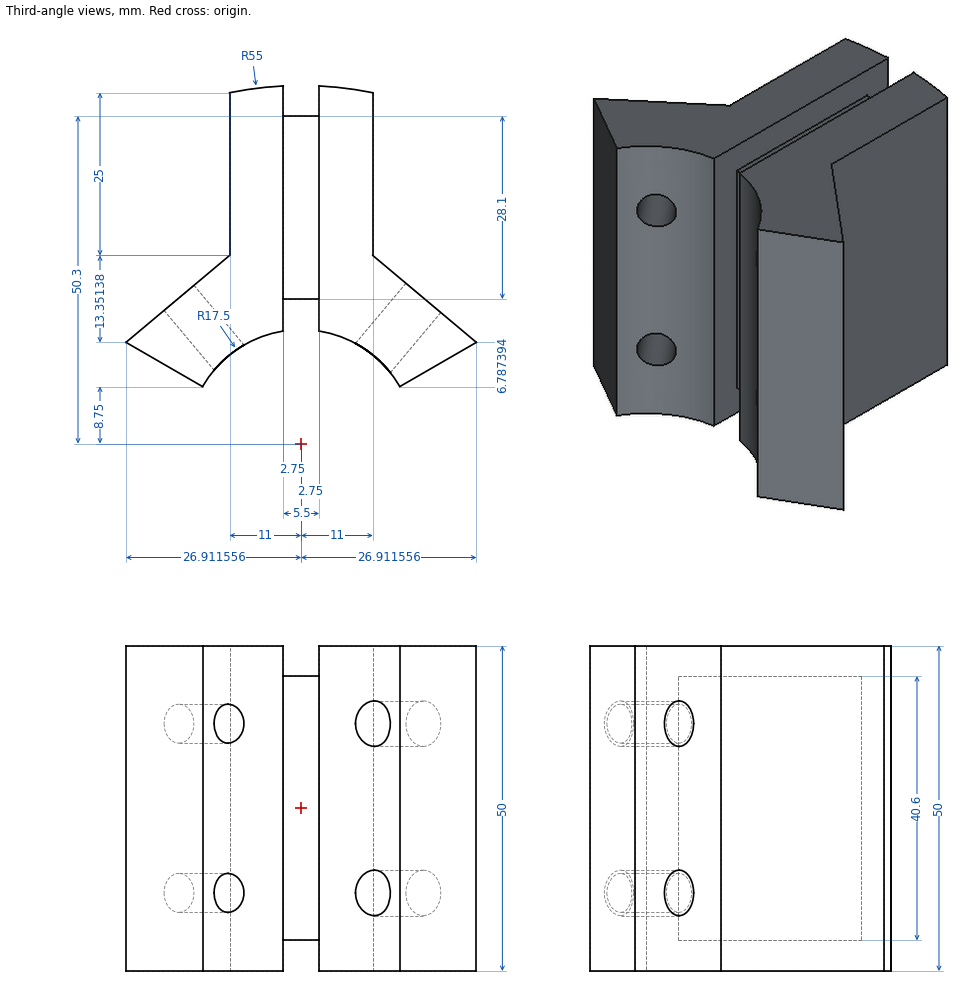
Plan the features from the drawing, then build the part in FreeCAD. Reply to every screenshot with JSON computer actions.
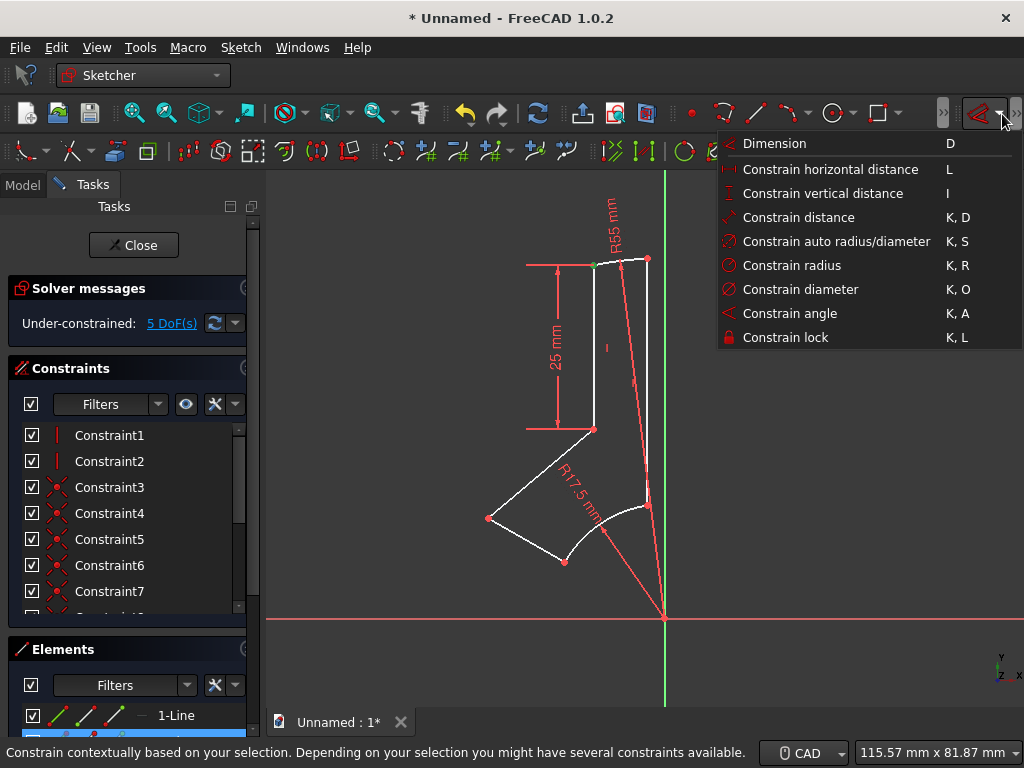
{"action": "left_click", "coordinate": [870, 169]}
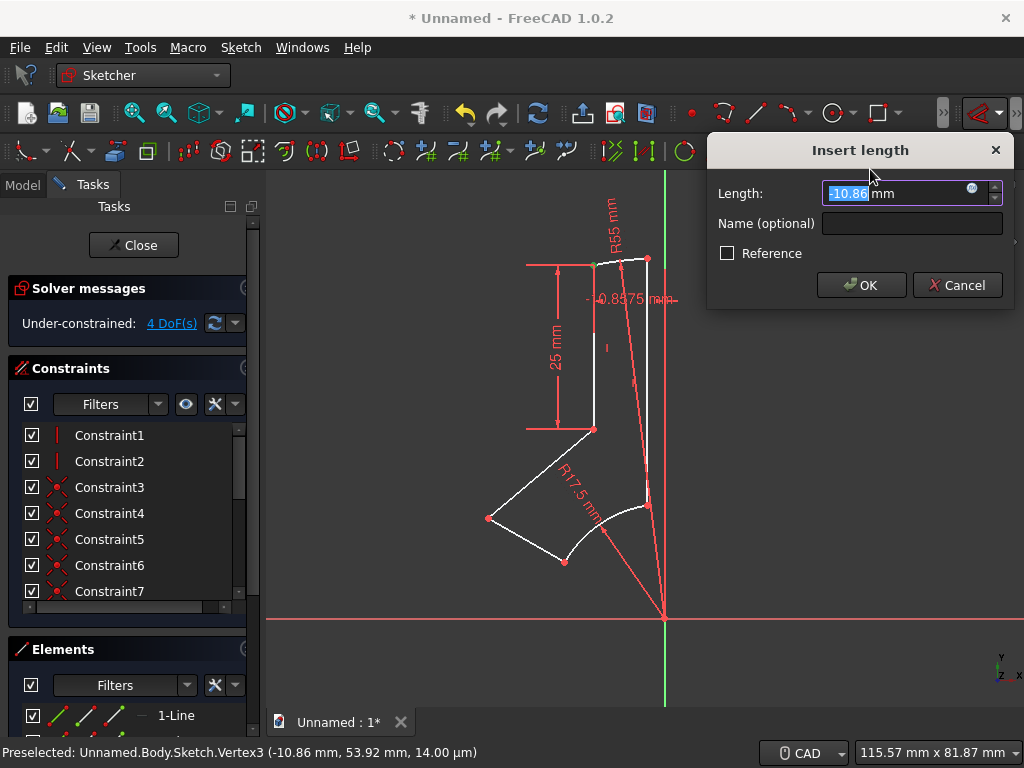
{"action": "type", "text": "-11"}
{"action": "key", "text": "Return"}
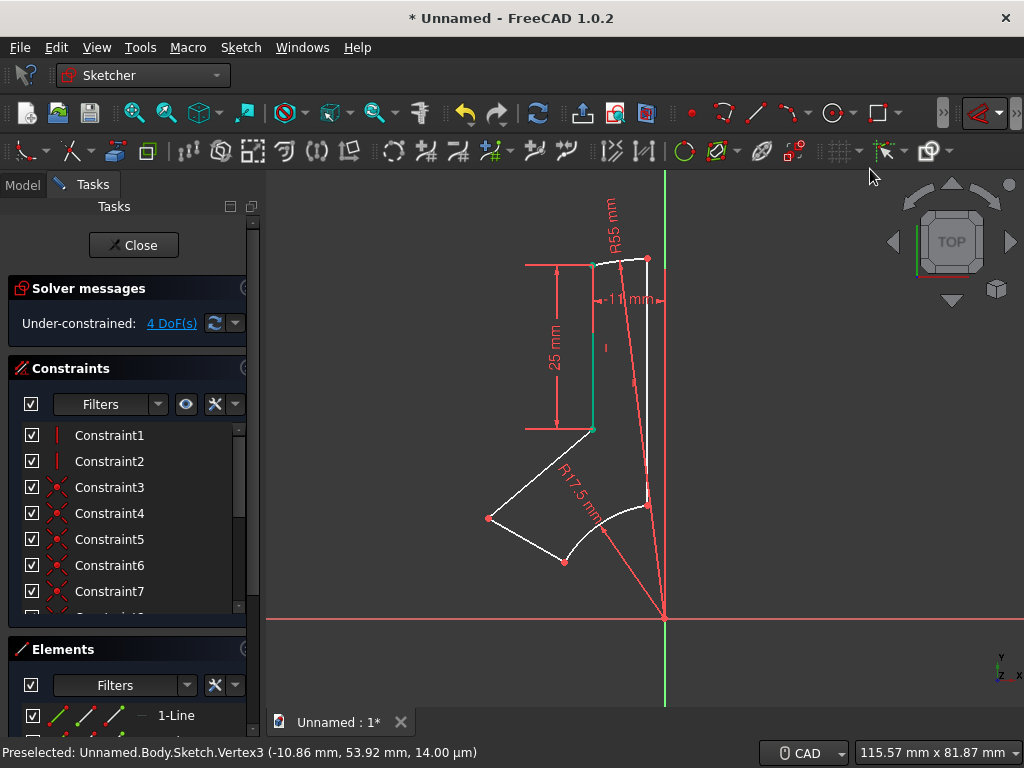
{"action": "scroll", "coordinate": [647, 506], "scroll_direction": "up", "scroll_amount": 4}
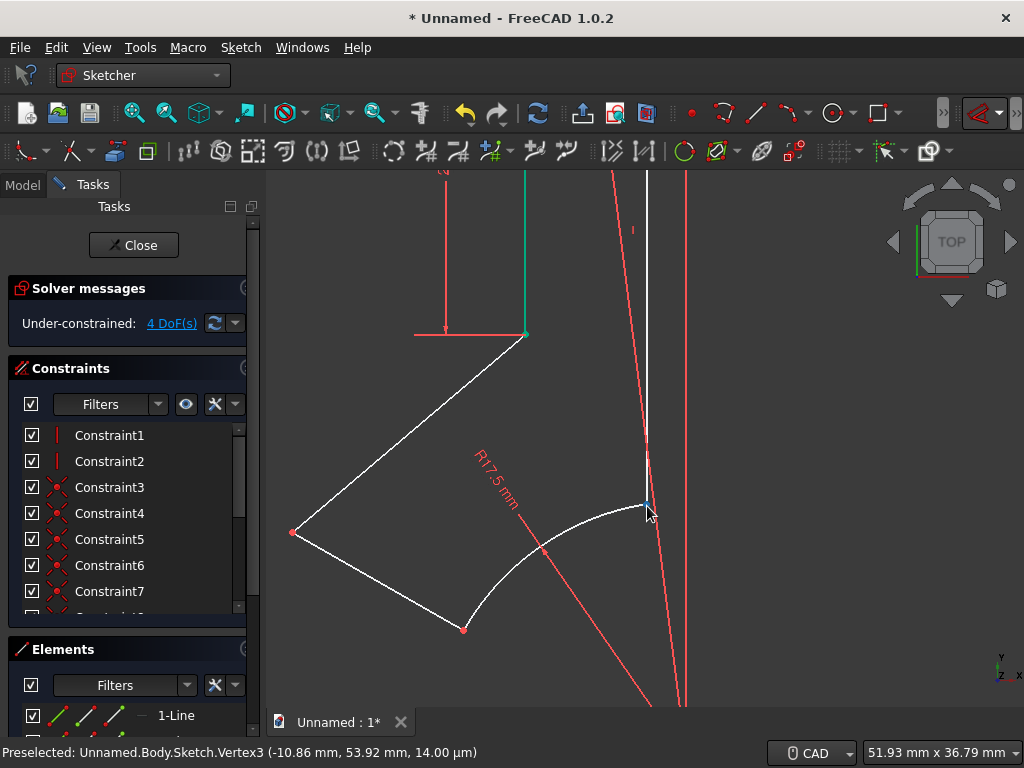
{"action": "left_click", "coordinate": [647, 504]}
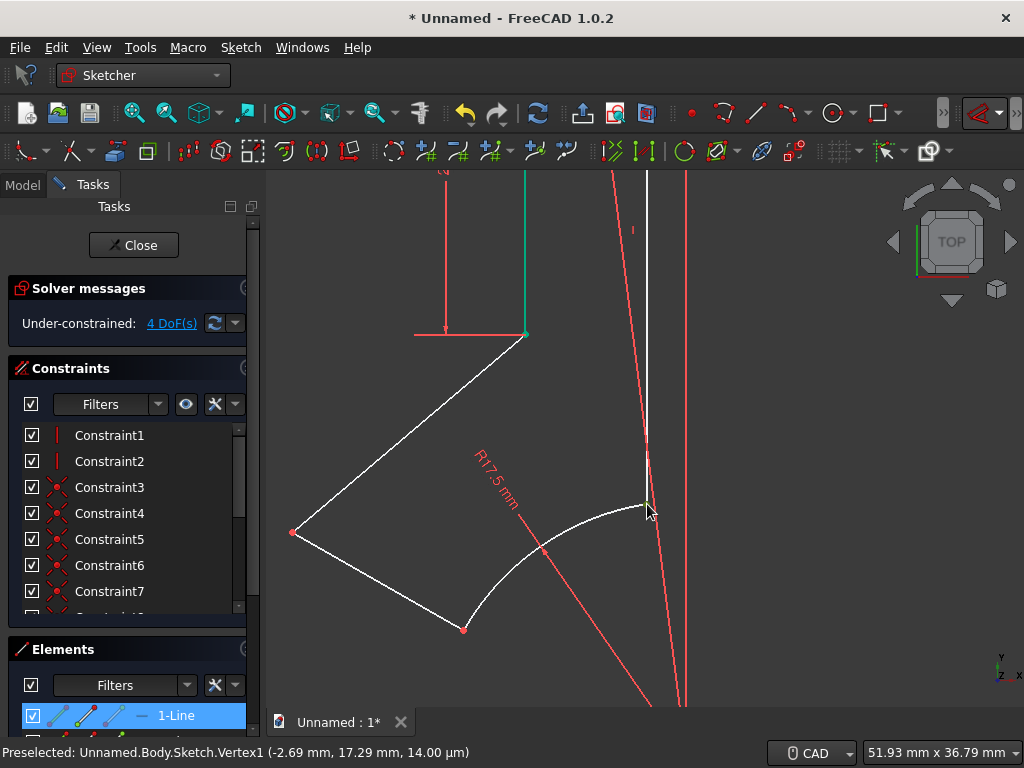
{"action": "key", "text": "l"}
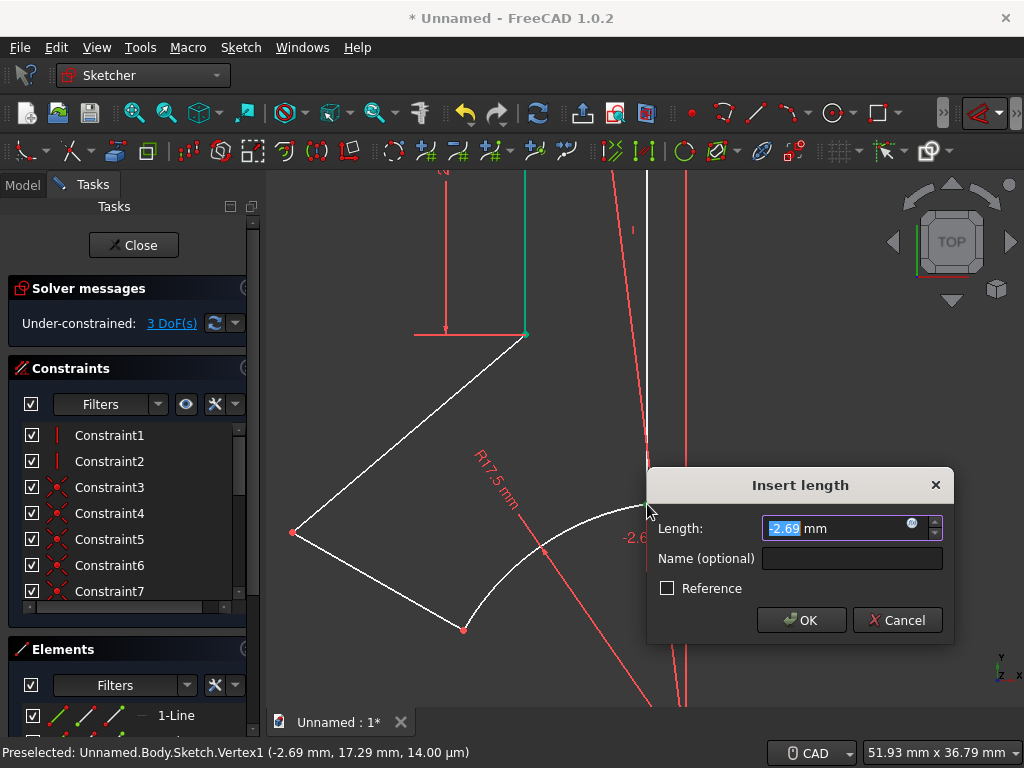
{"action": "type", "text": "-2.75"}
{"action": "key", "text": "Return"}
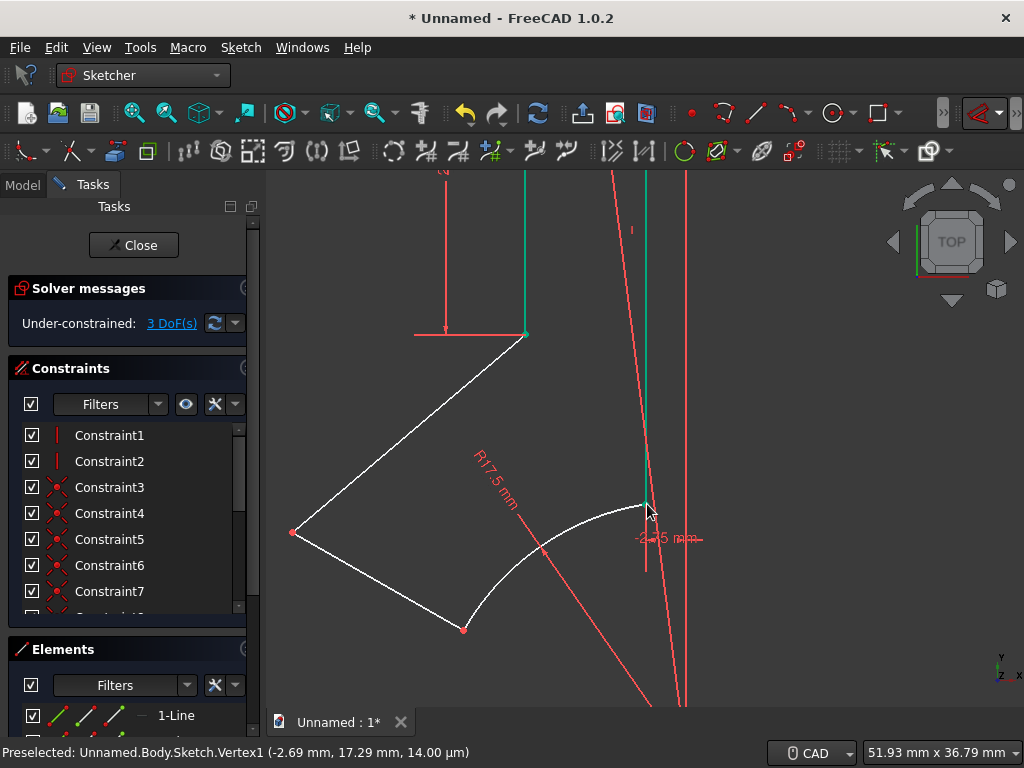
{"action": "left_click", "coordinate": [464, 631]}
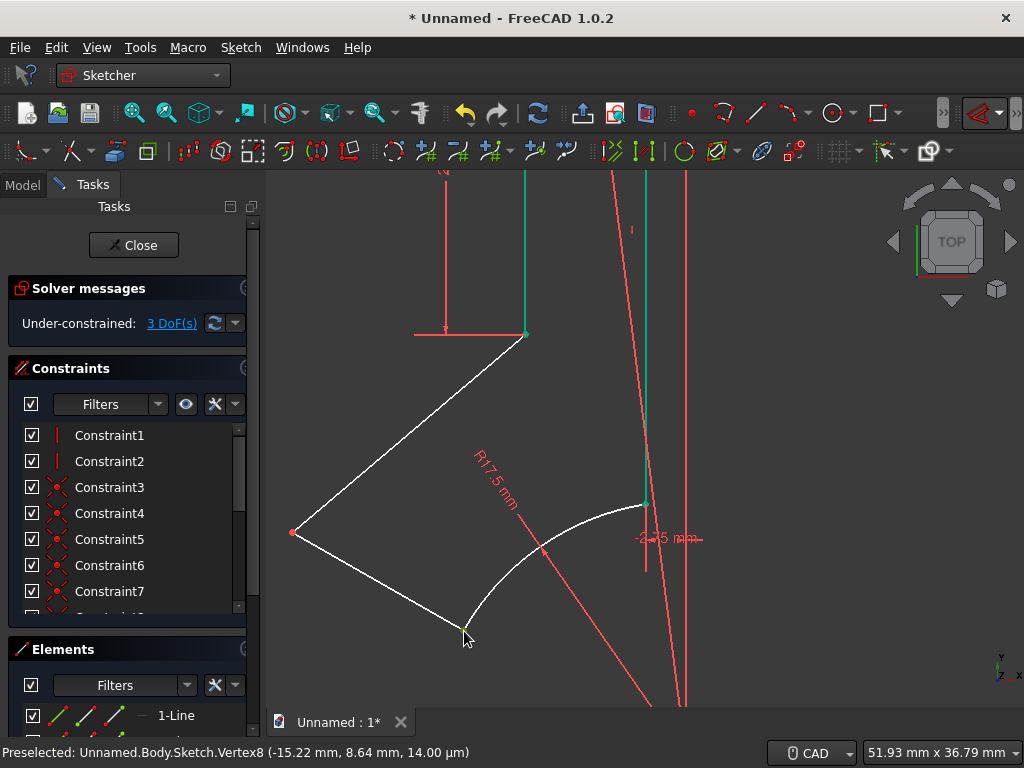
{"action": "key", "text": "i"}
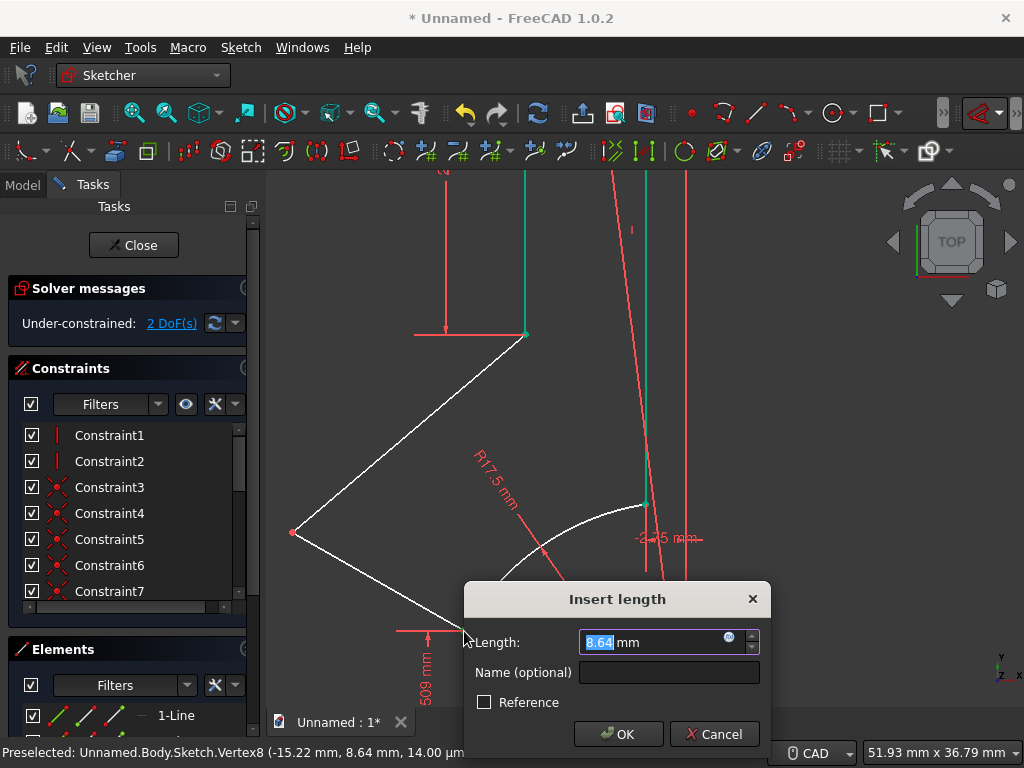
{"action": "type", "text": "8.75"}
{"action": "key", "text": "Return"}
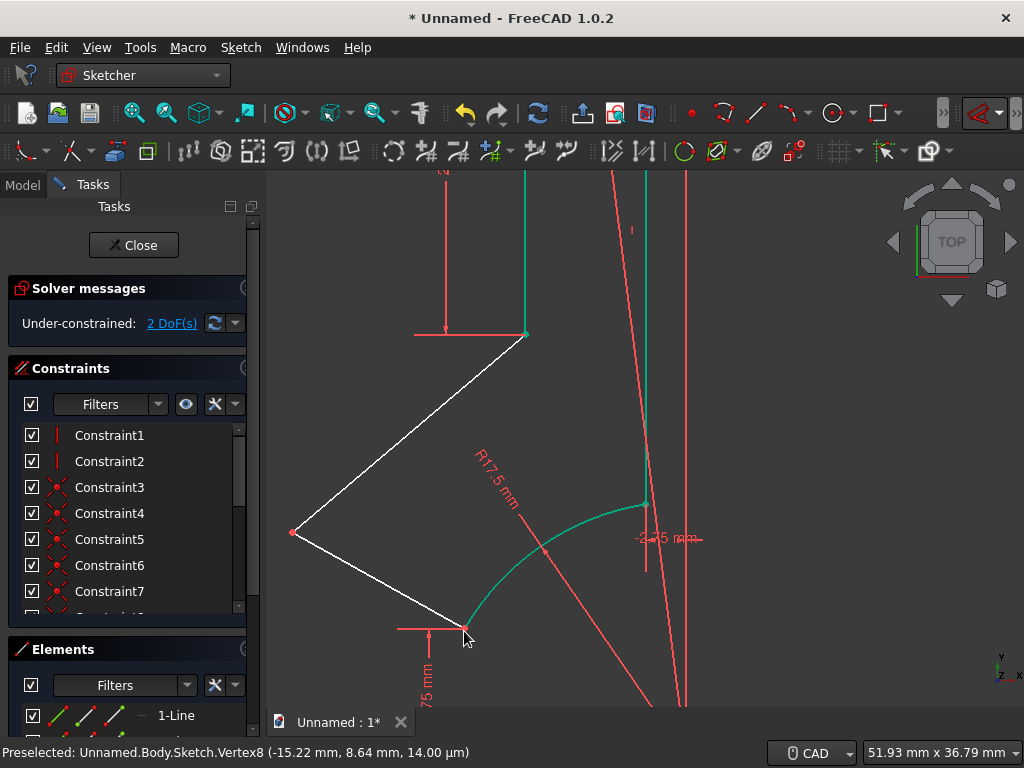
{"action": "left_click", "coordinate": [456, 394]}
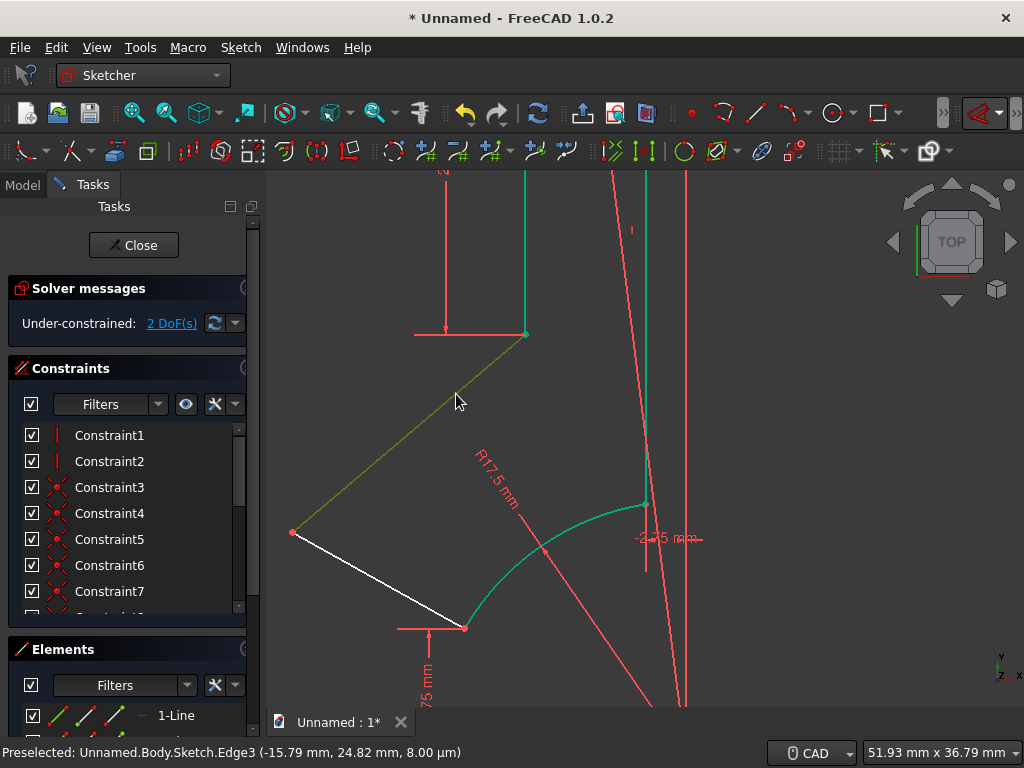
{"action": "left_click", "coordinate": [1002, 114]}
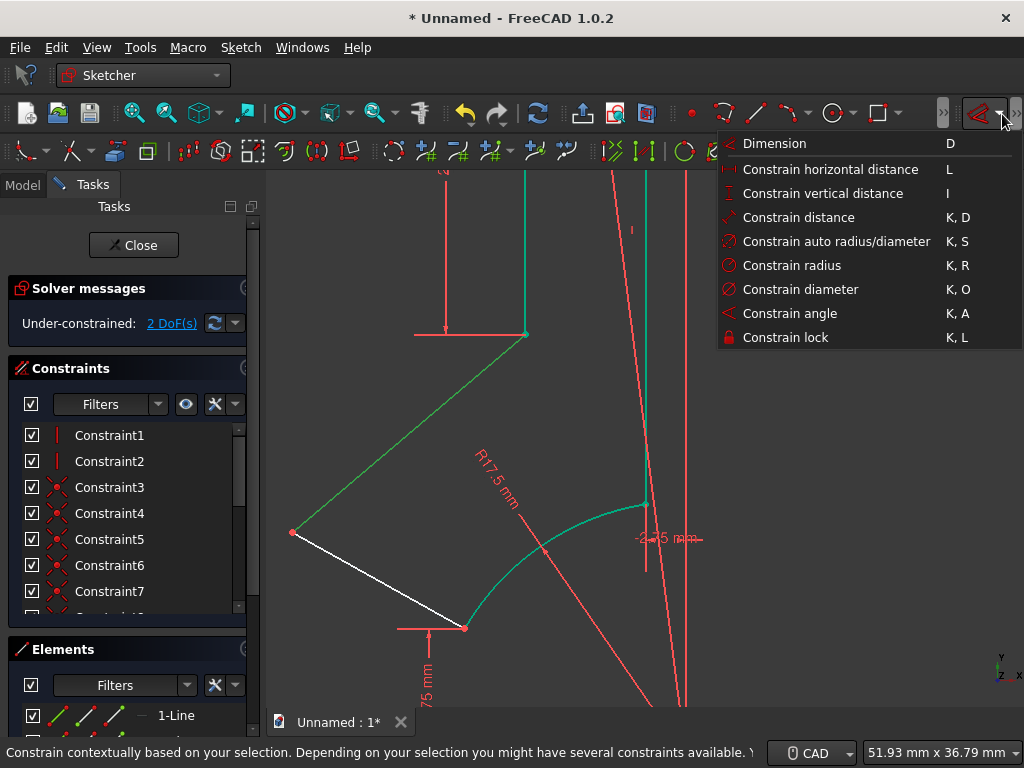
{"action": "left_click", "coordinate": [870, 193]}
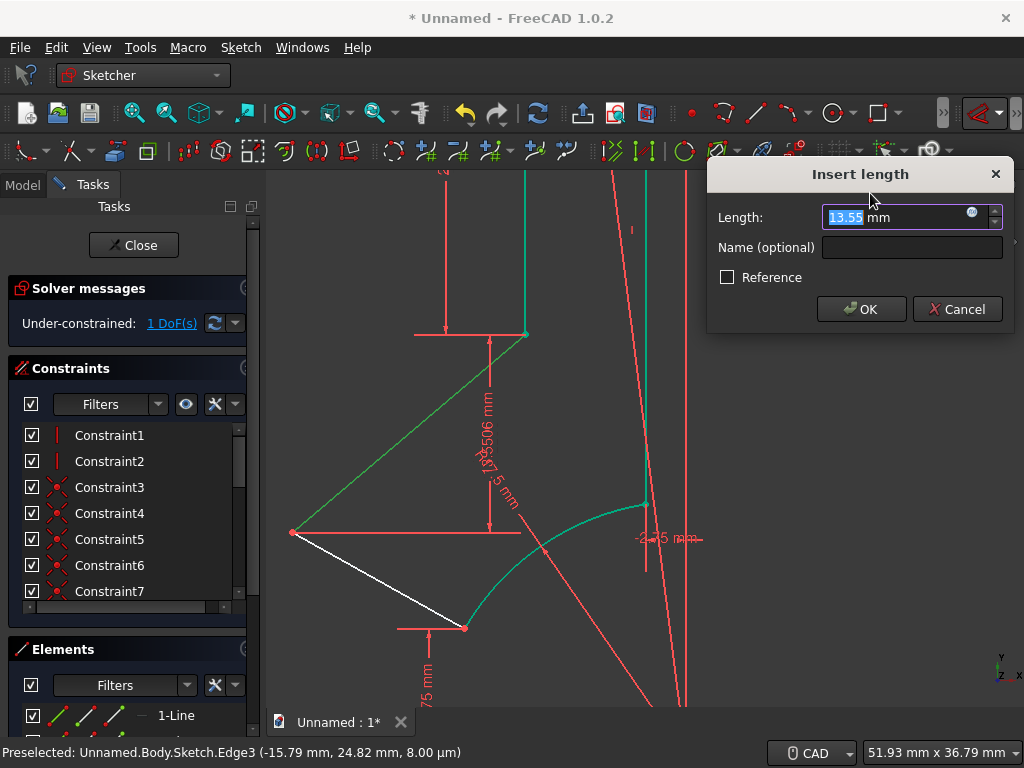
{"action": "type", "text": "13.35138"}
{"action": "key", "text": "Return"}